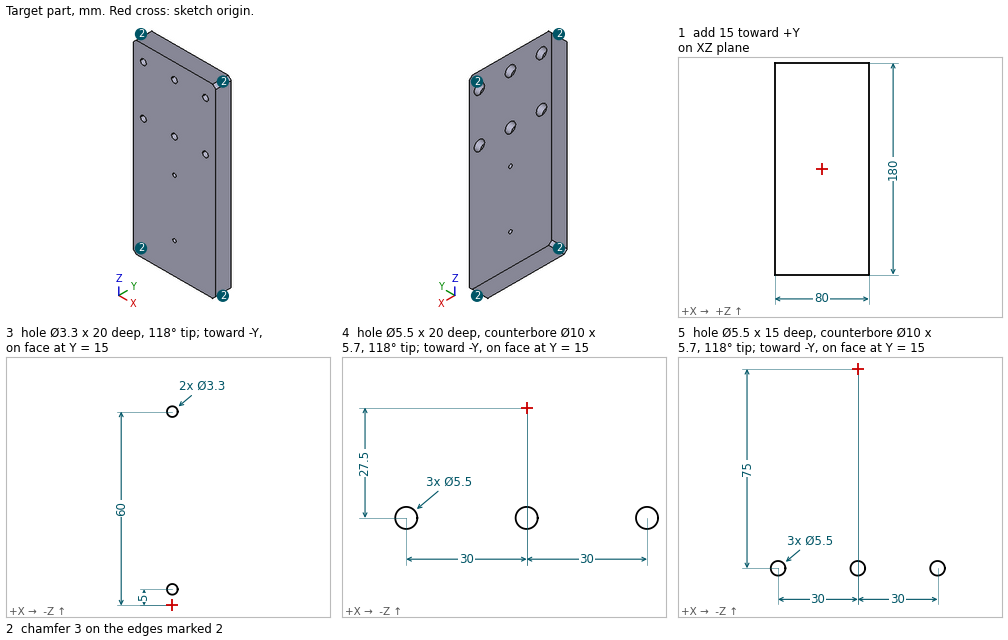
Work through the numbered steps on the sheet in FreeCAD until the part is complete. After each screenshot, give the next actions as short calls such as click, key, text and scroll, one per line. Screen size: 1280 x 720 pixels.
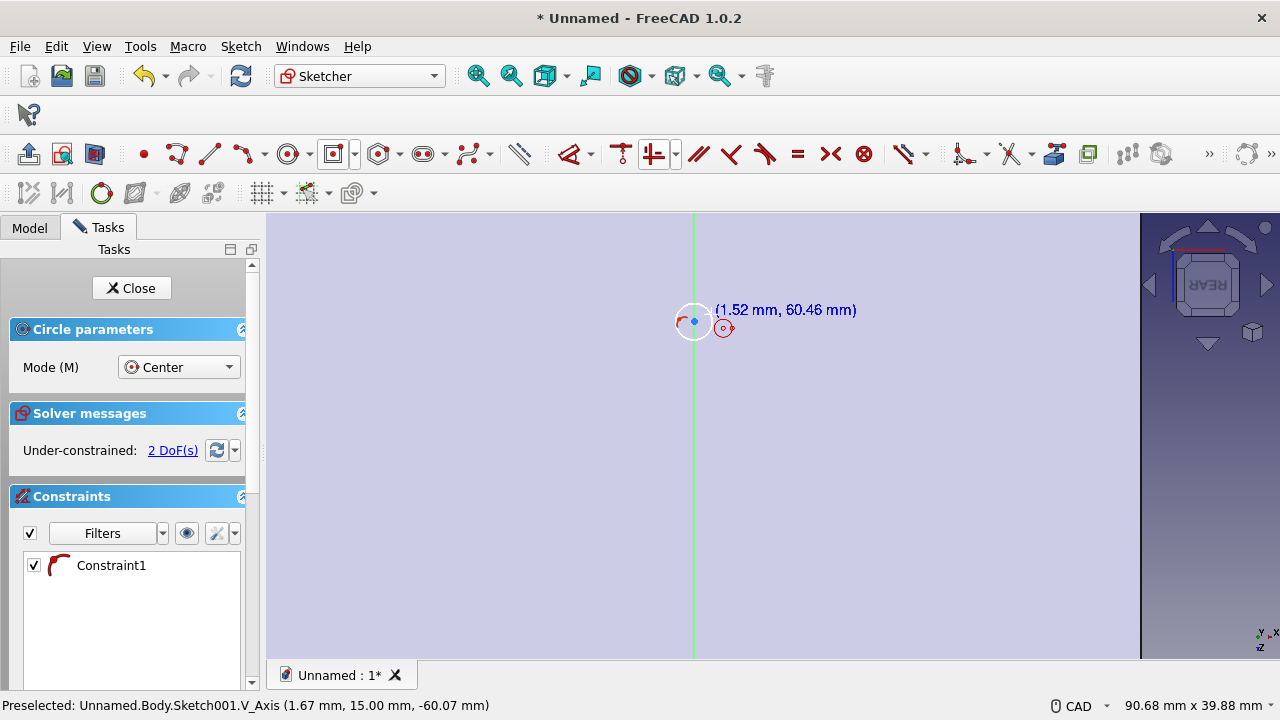
scroll(711, 314, down, 5)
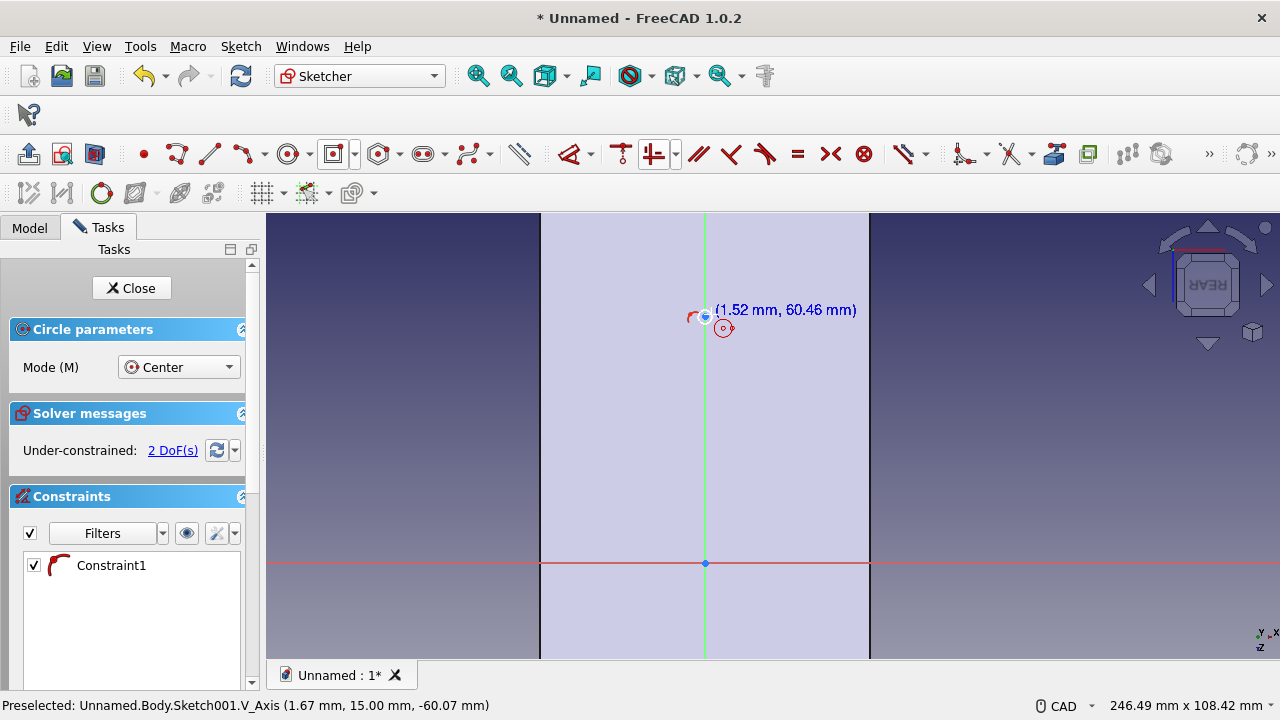
scroll(705, 543, up, 7)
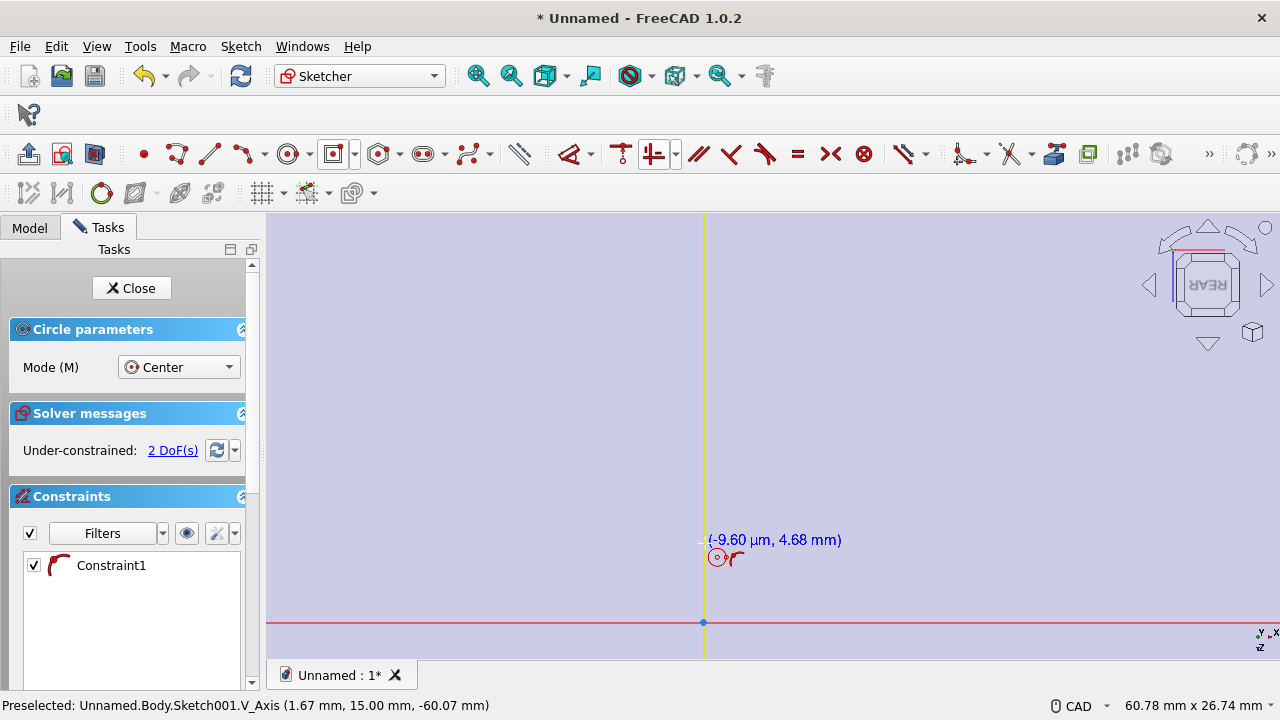
scroll(705, 543, down, 7)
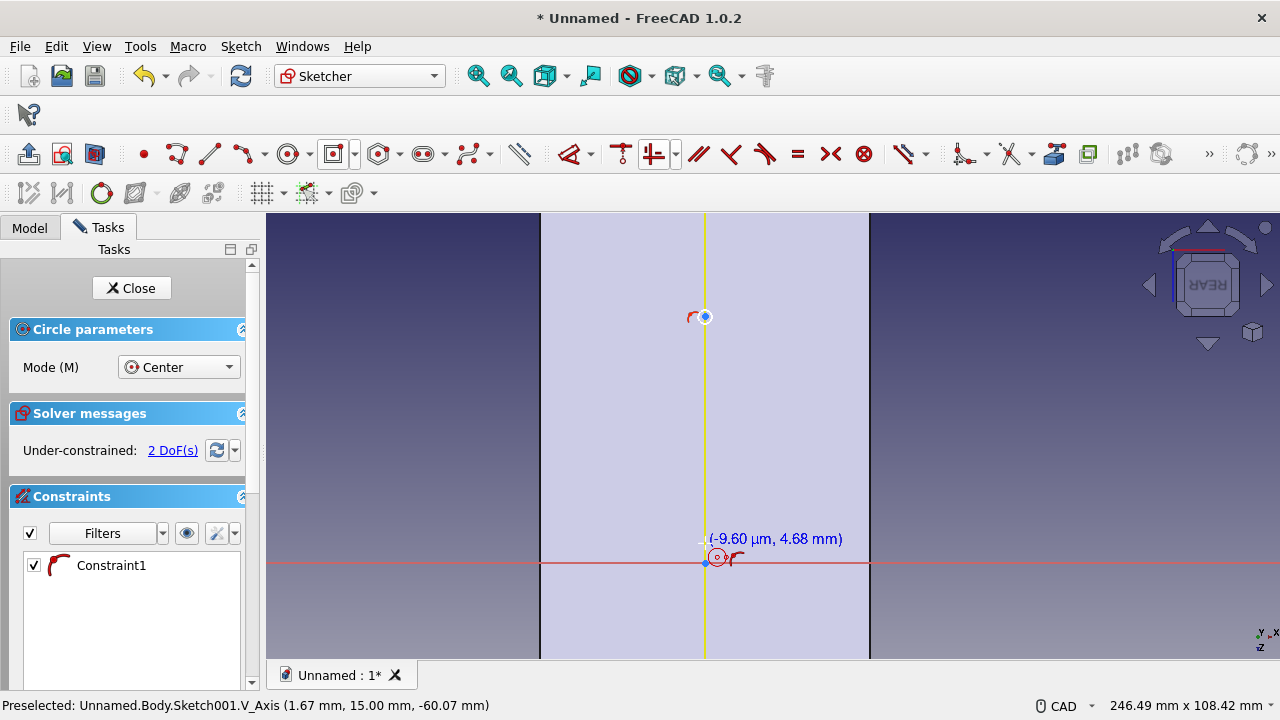
click(705, 543)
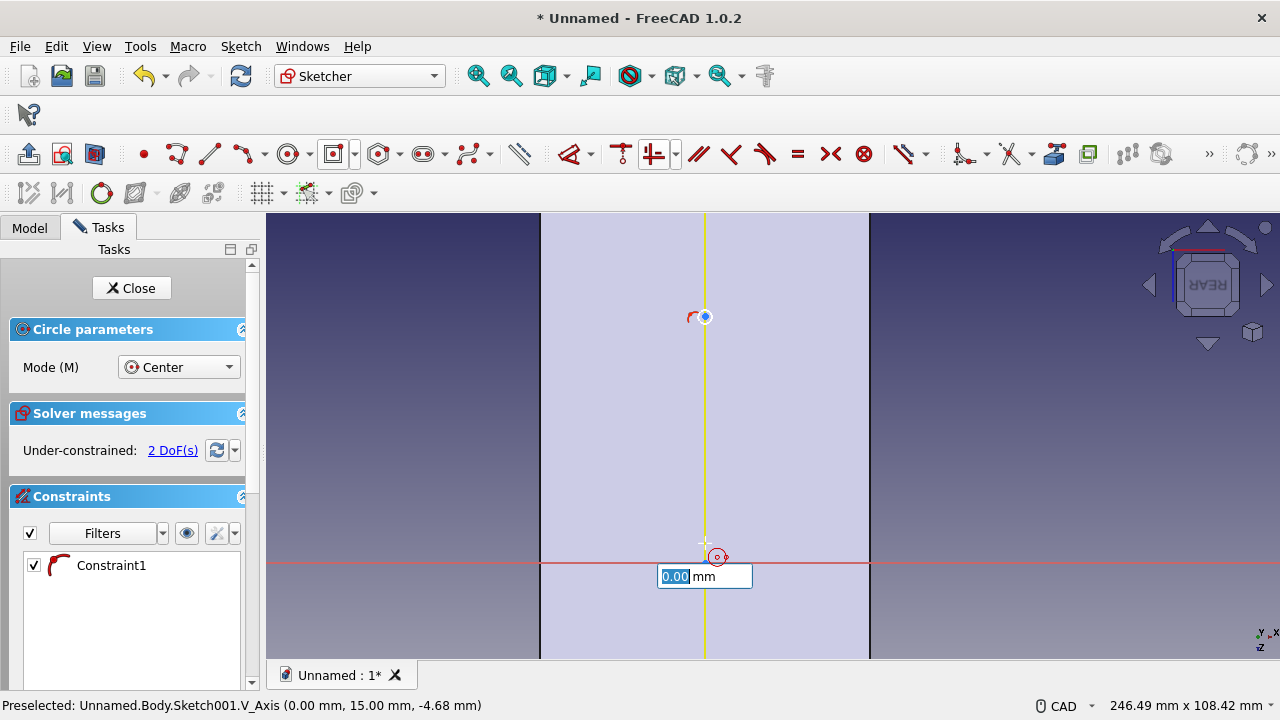
scroll(711, 540, up, 5)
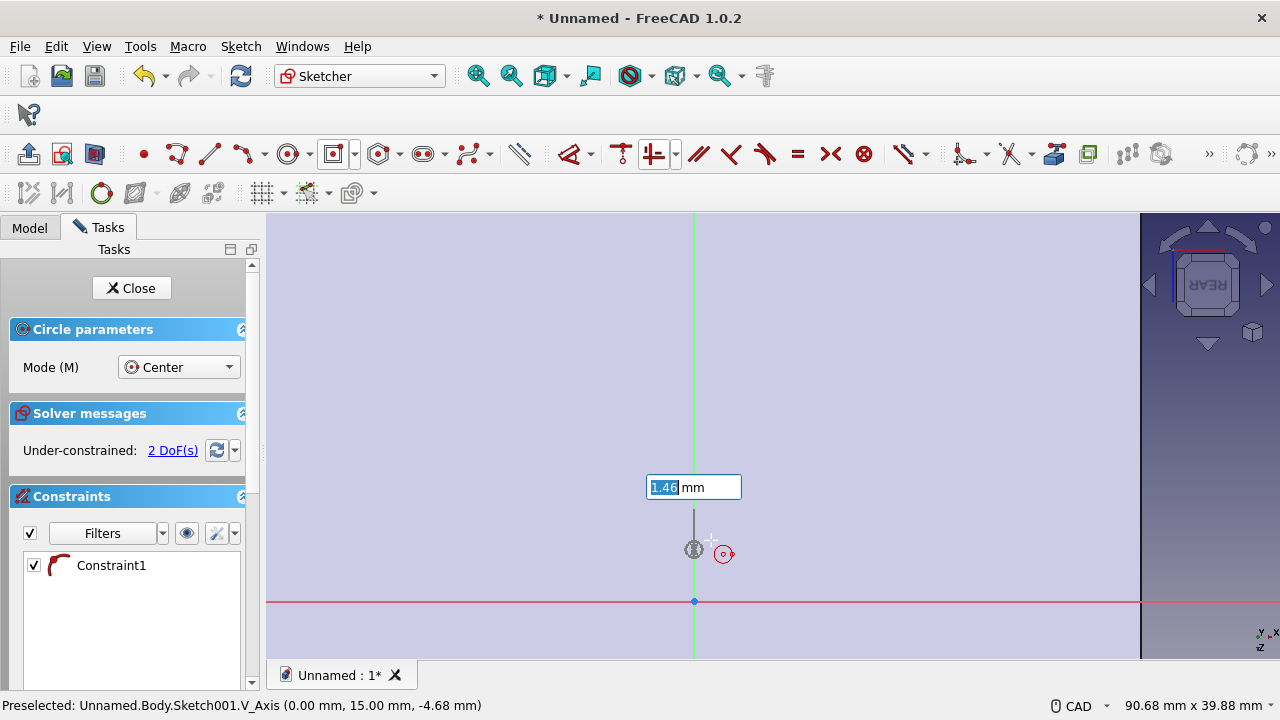
click(711, 540)
key(Escape)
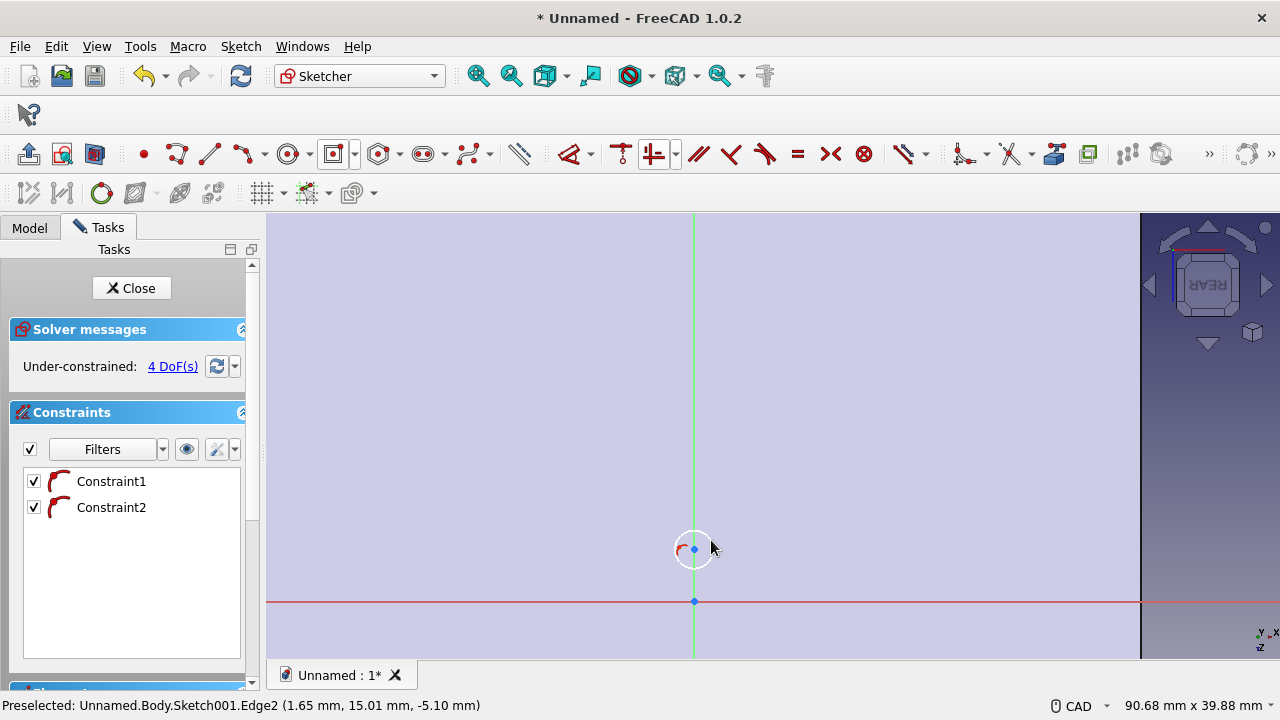
scroll(711, 540, down, 5)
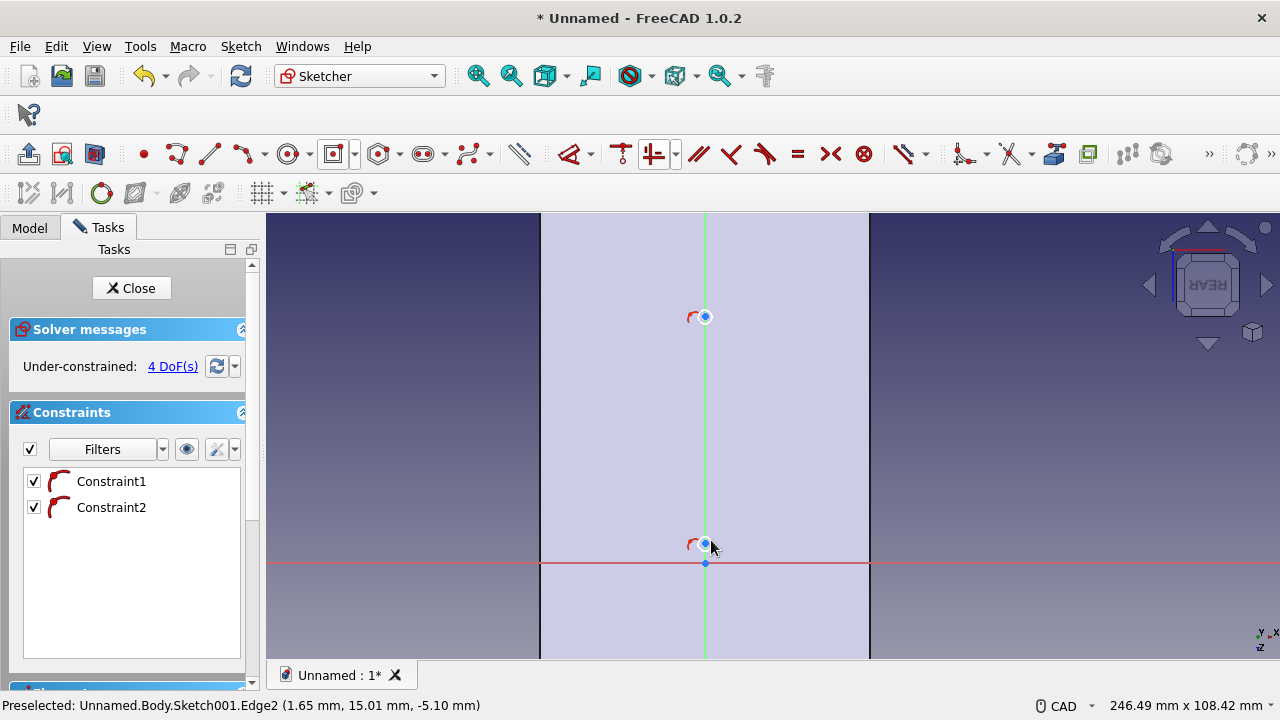
scroll(710, 312, up, 6)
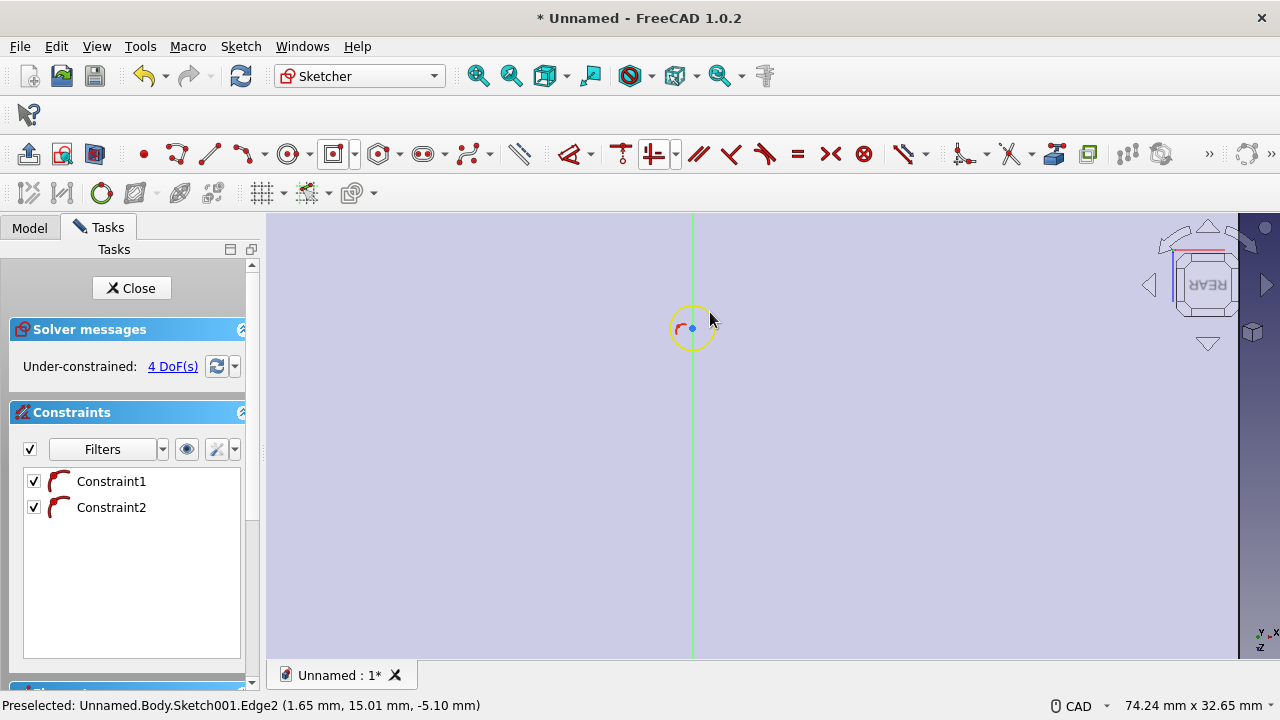
click(708, 312)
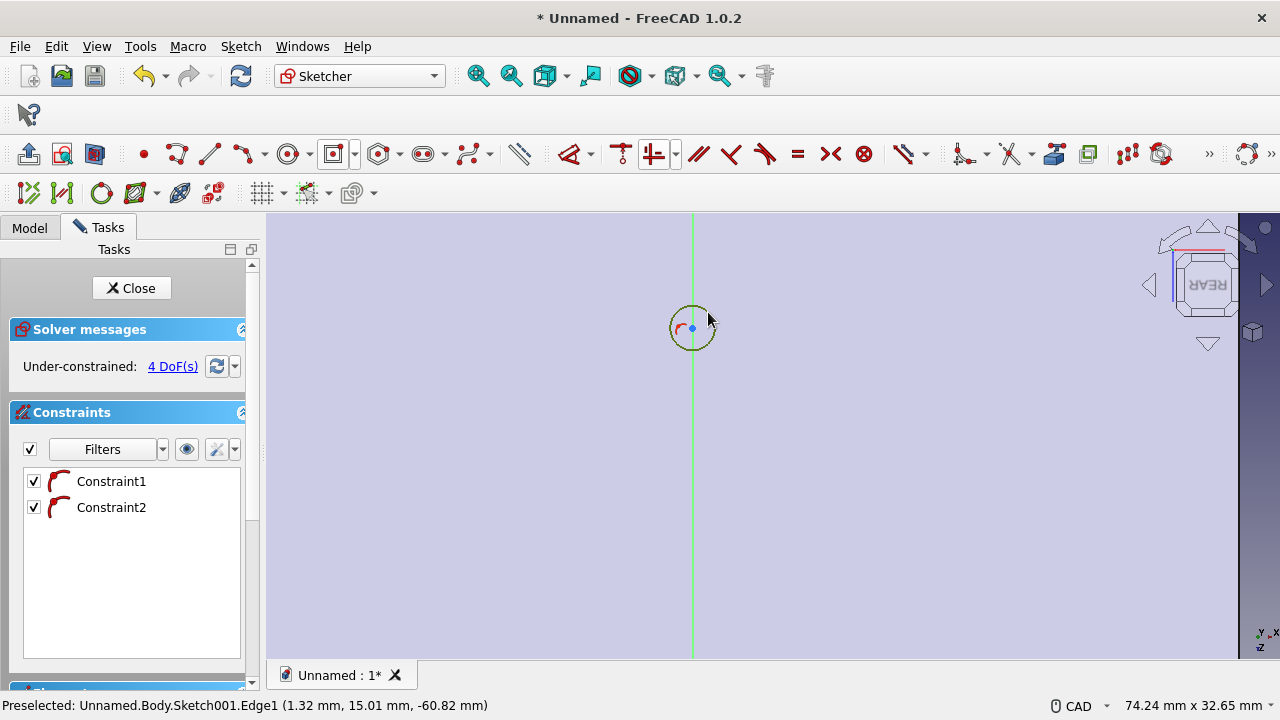
scroll(710, 312, down, 6)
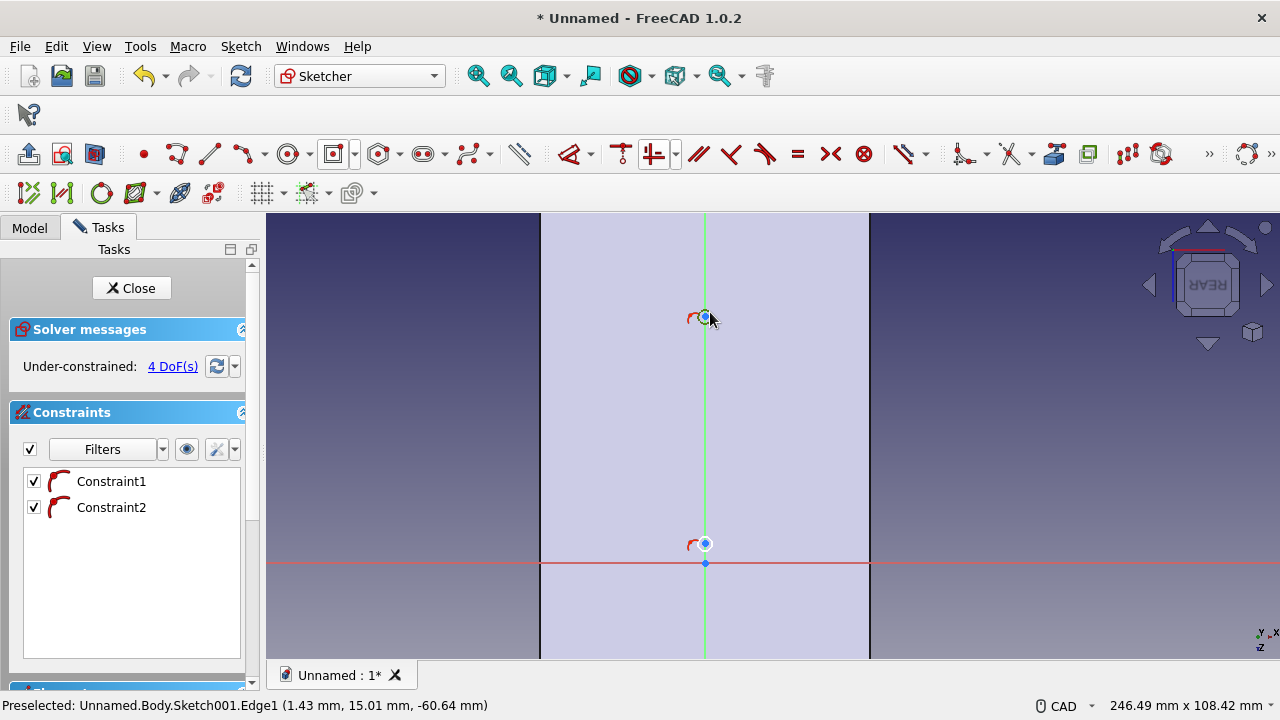
scroll(710, 539, up, 6)